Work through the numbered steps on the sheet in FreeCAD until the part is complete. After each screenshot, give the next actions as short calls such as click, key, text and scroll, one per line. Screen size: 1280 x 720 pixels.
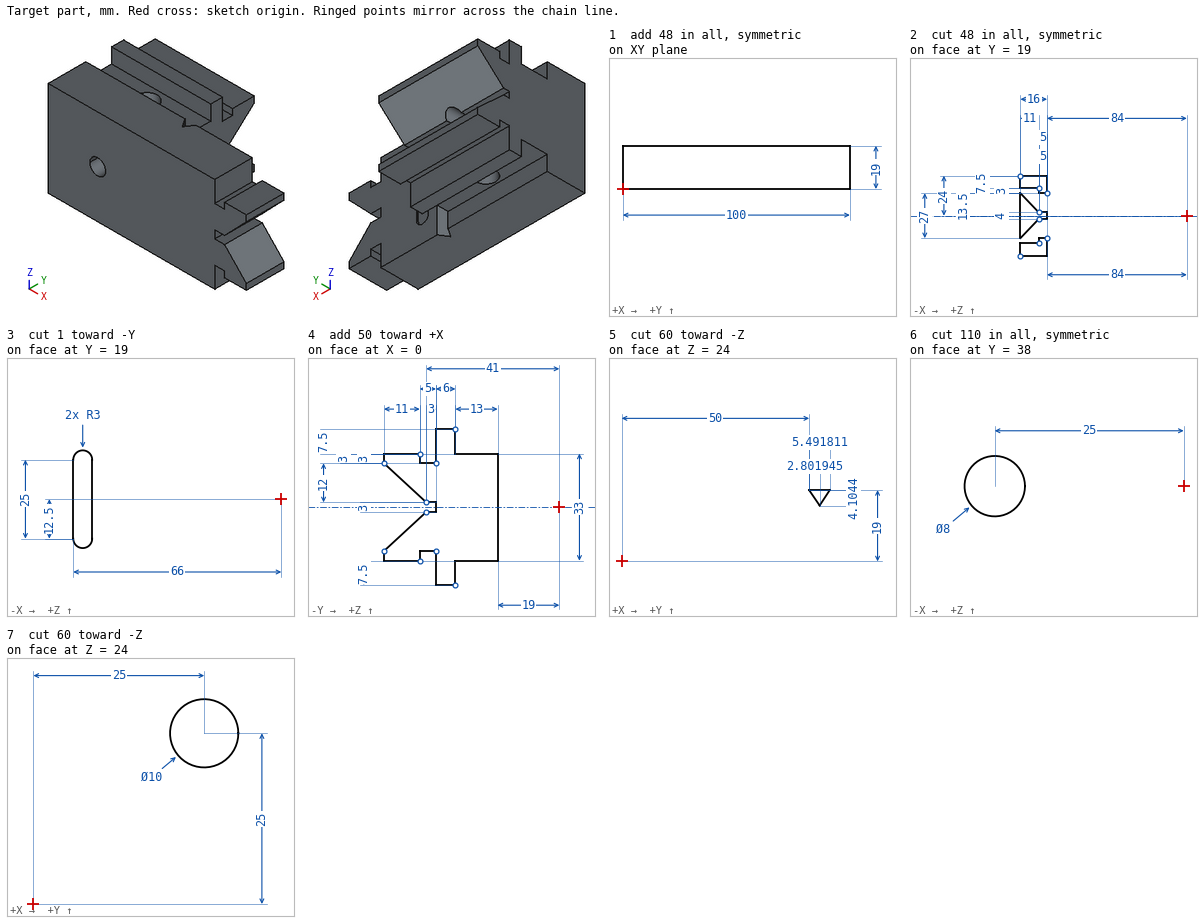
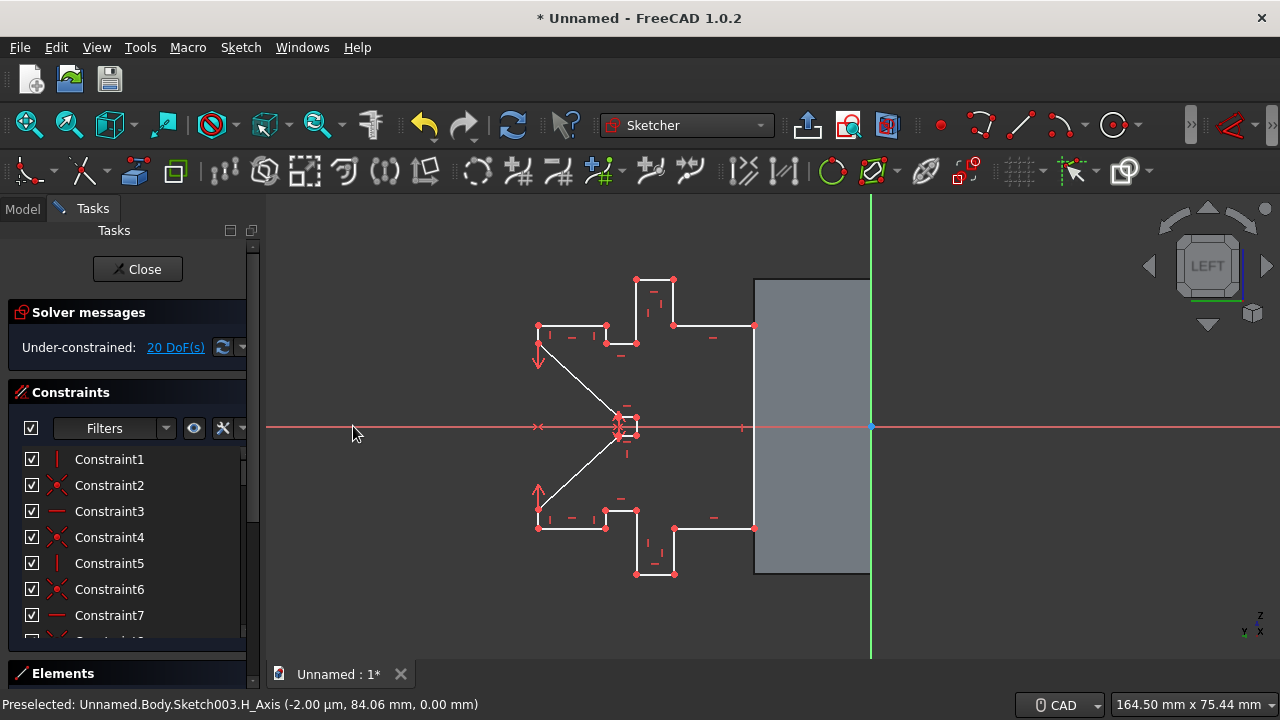
click(606, 326)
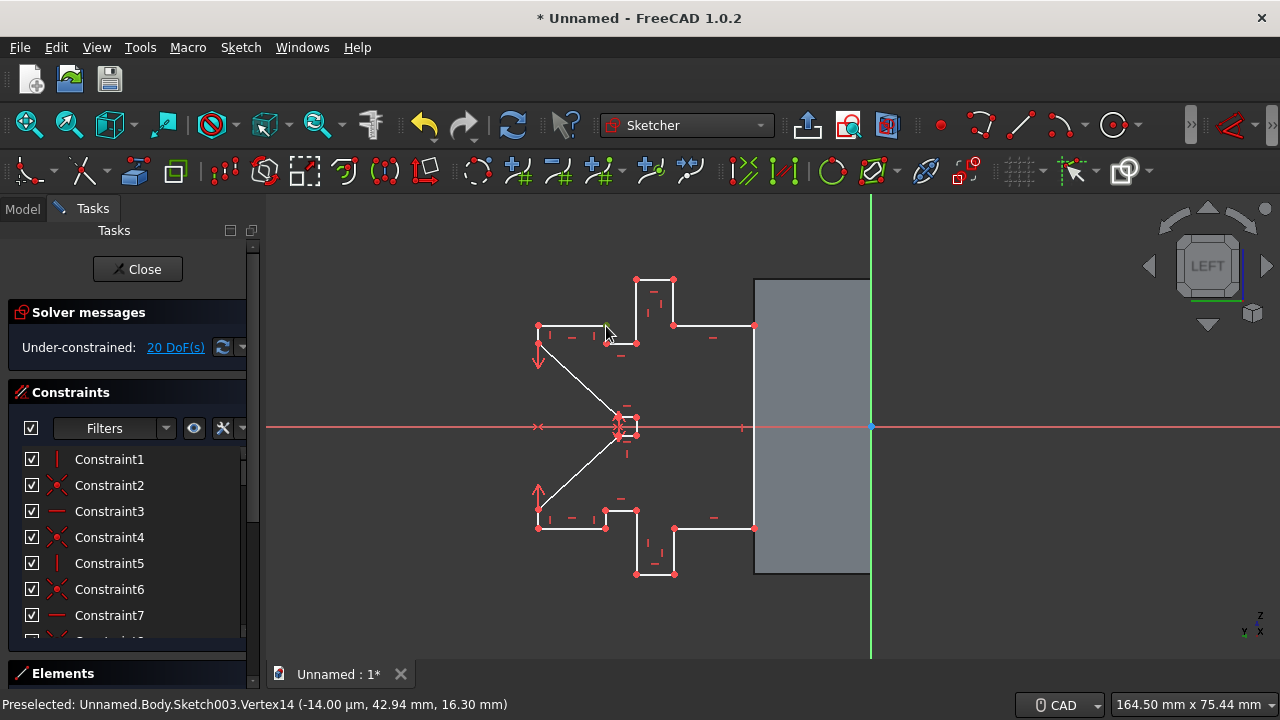
click(606, 529)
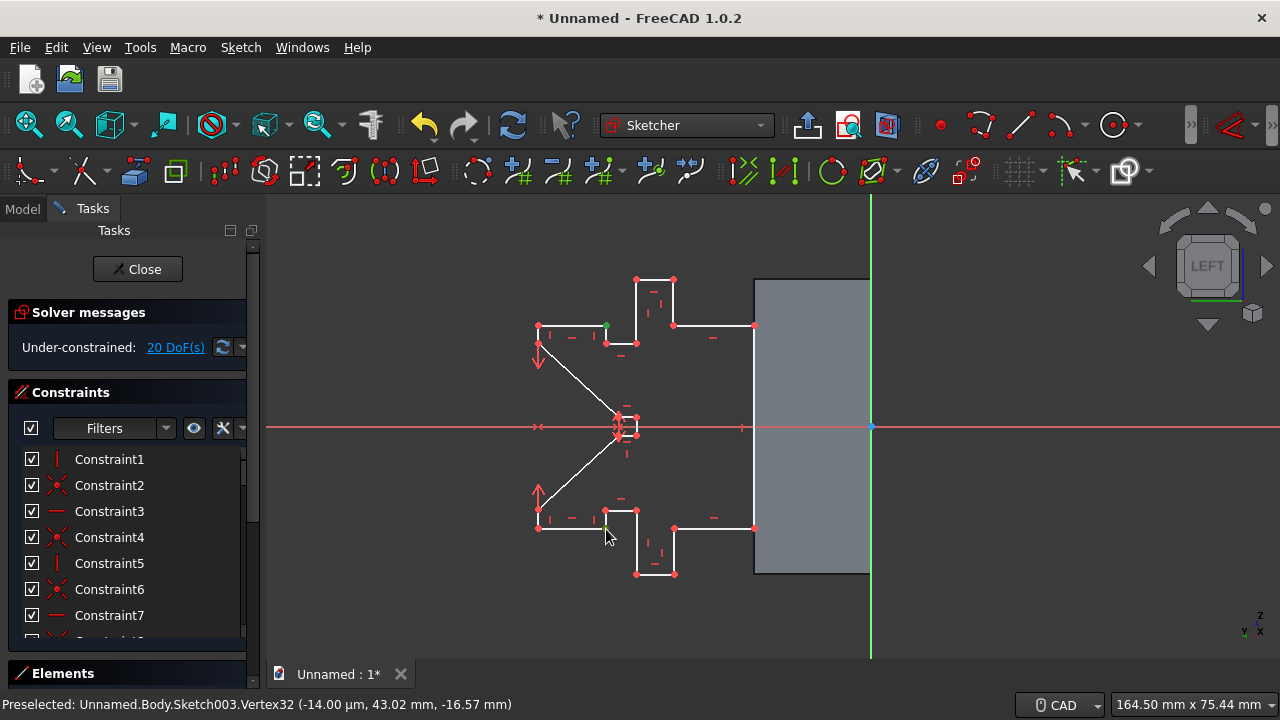
click(353, 426)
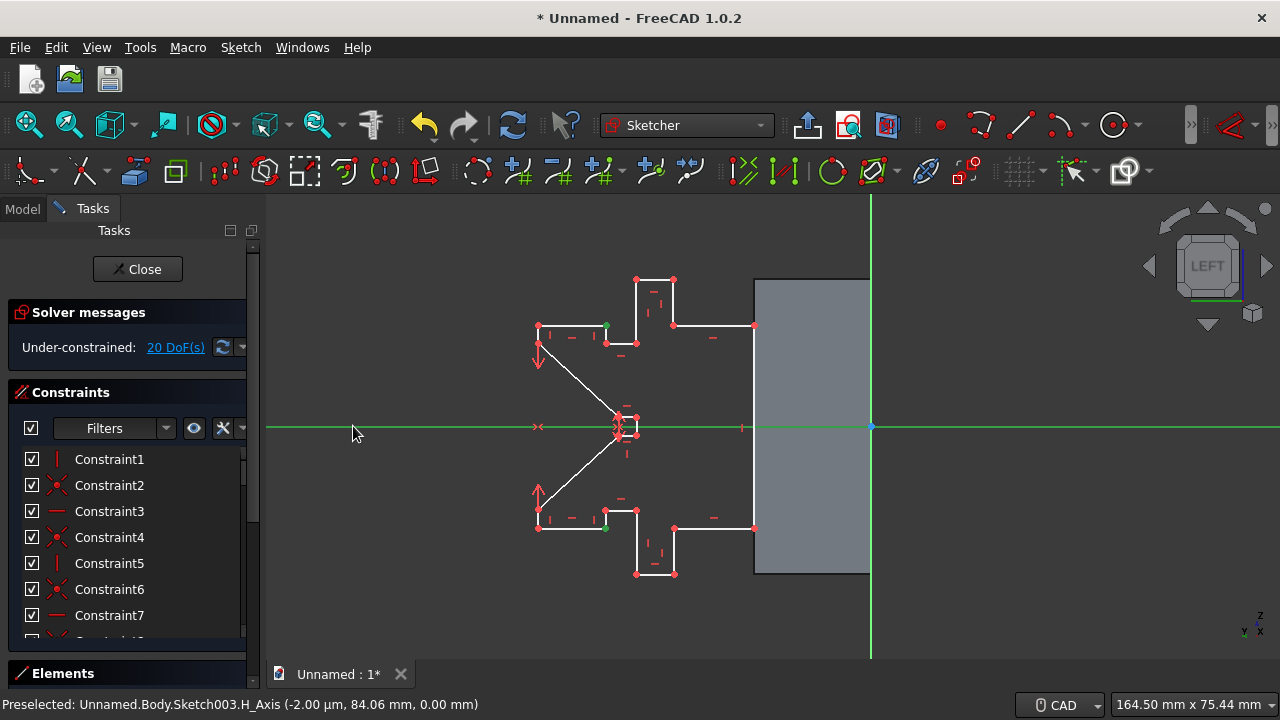
key(s)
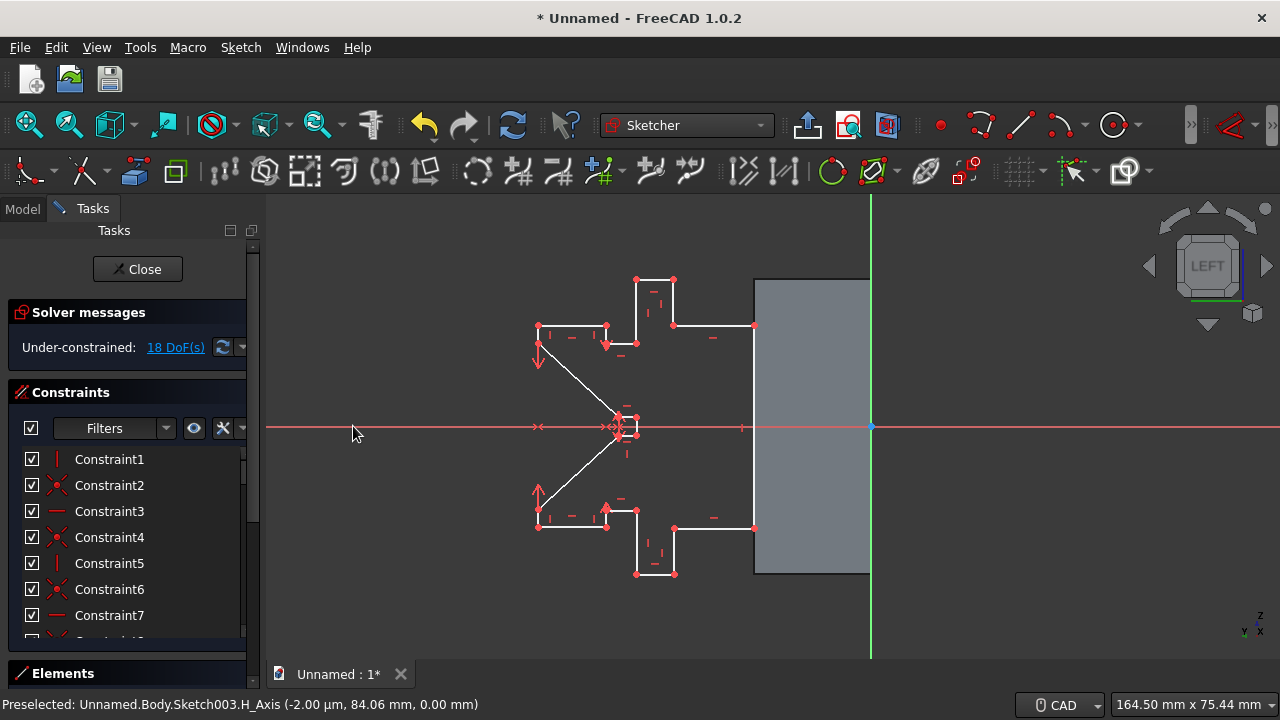
click(636, 344)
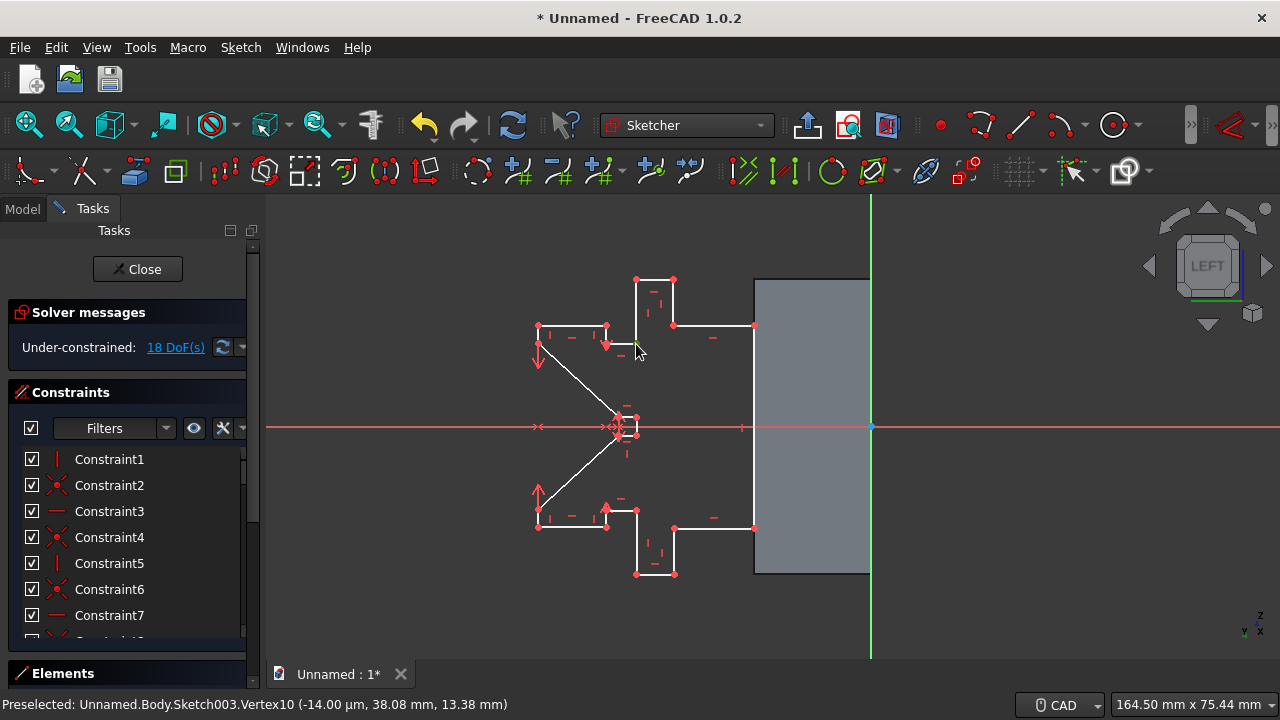
click(637, 511)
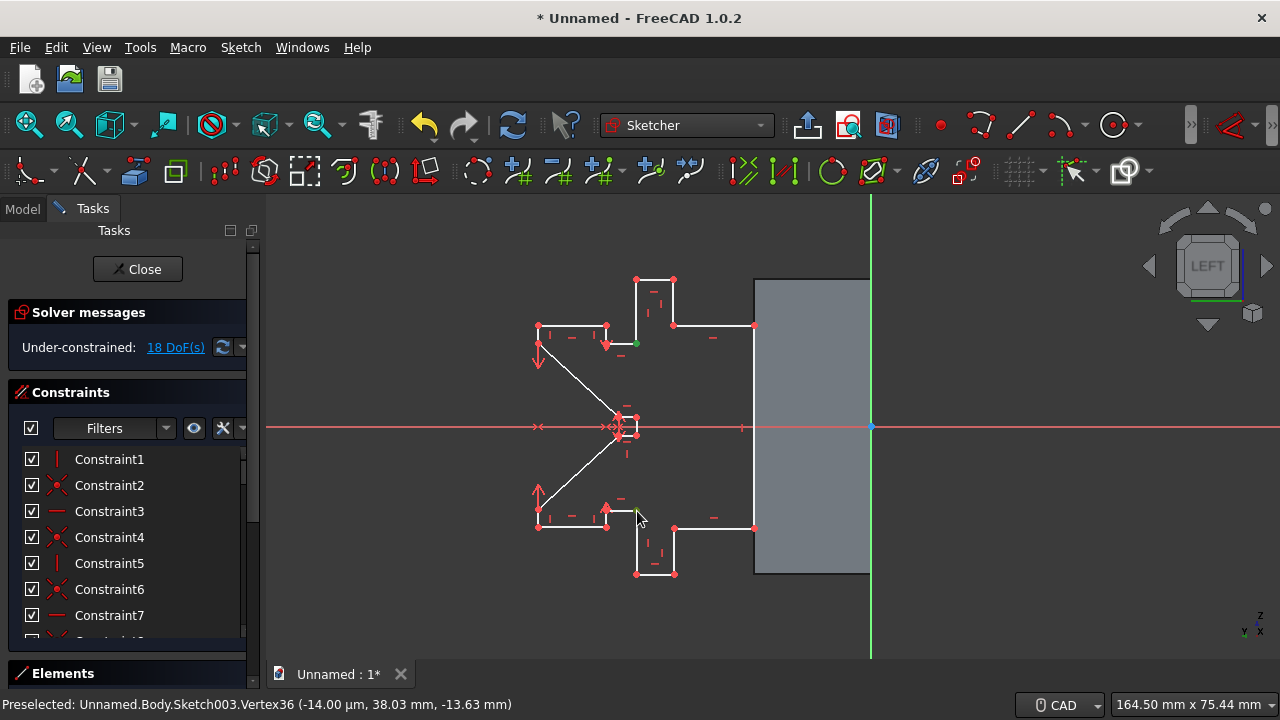
click(353, 426)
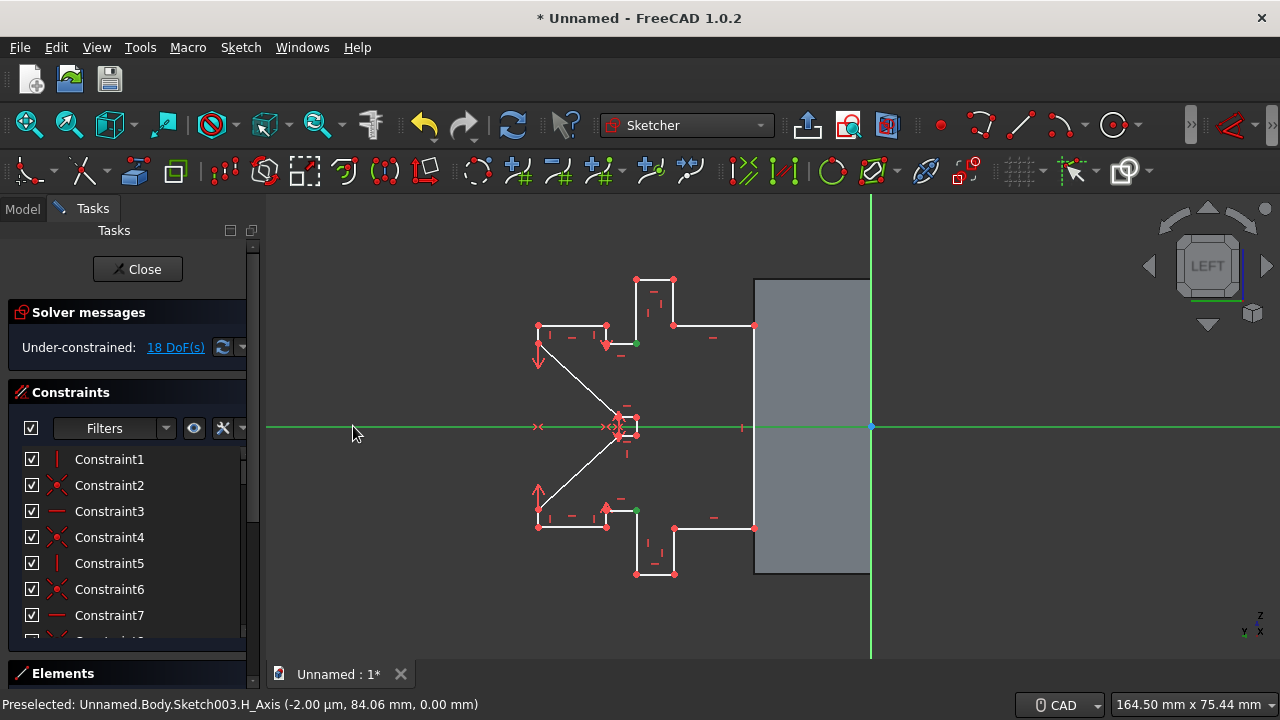
key(s)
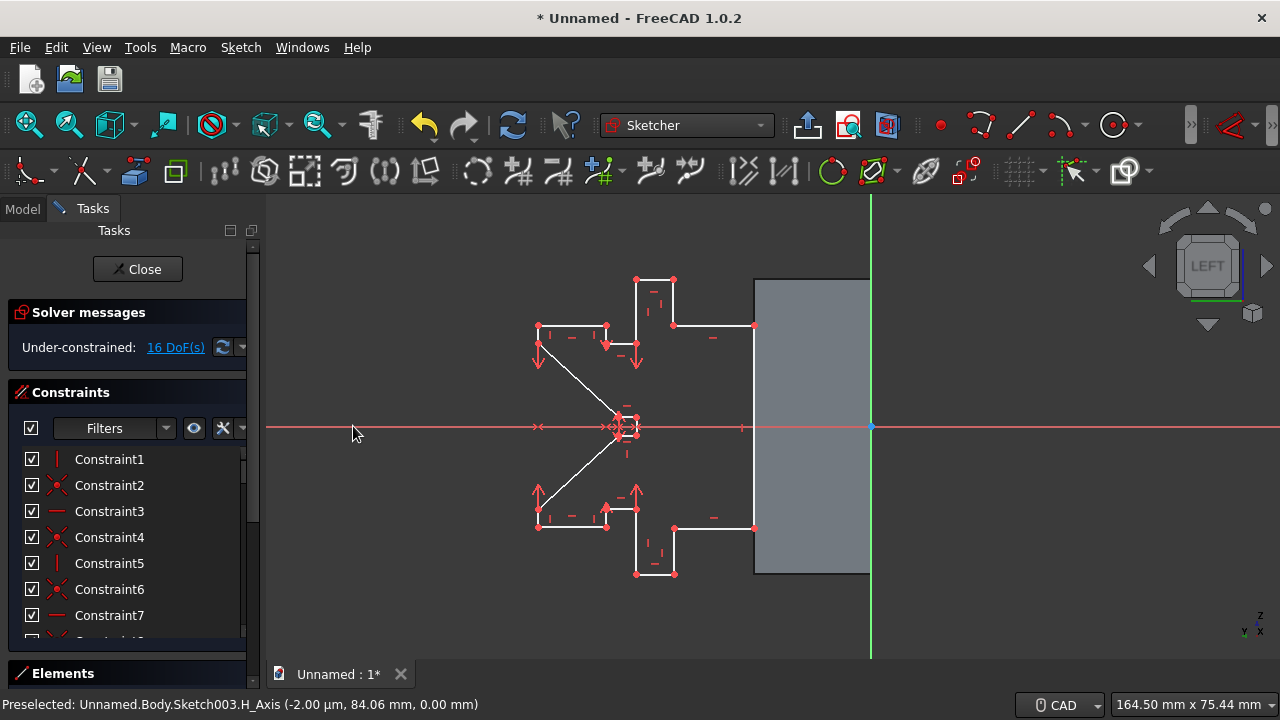
click(673, 280)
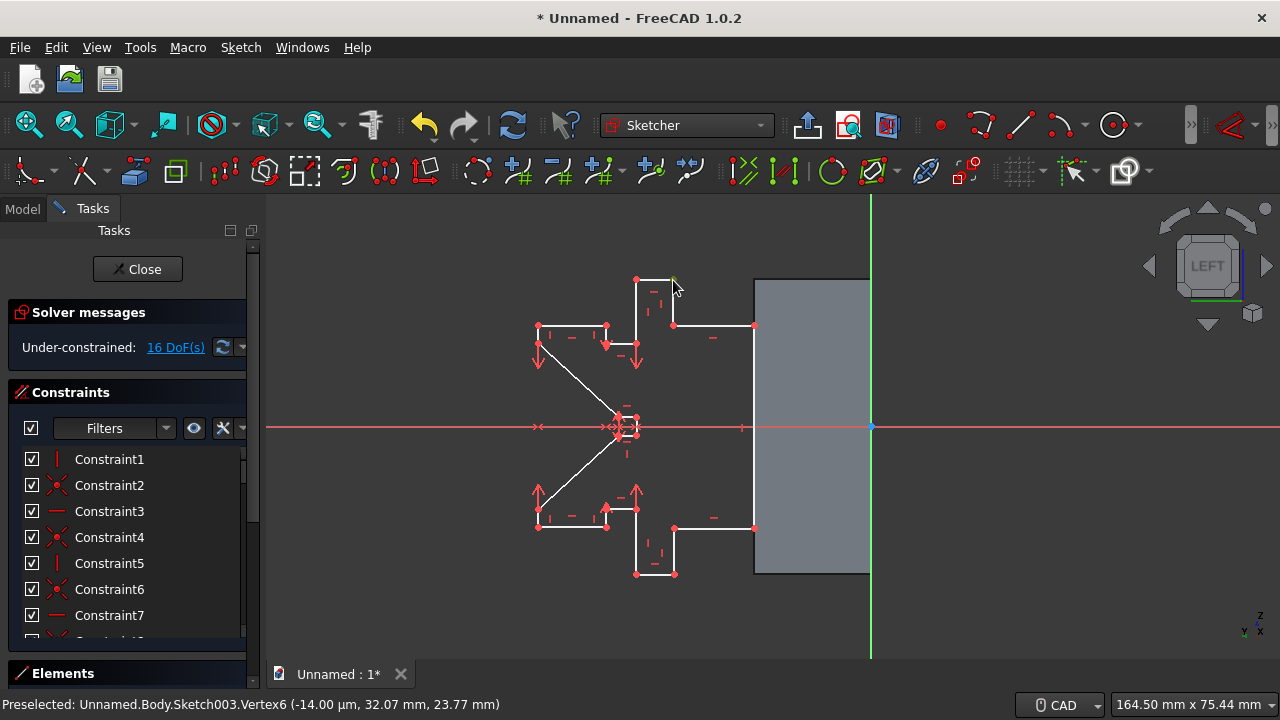
click(674, 575)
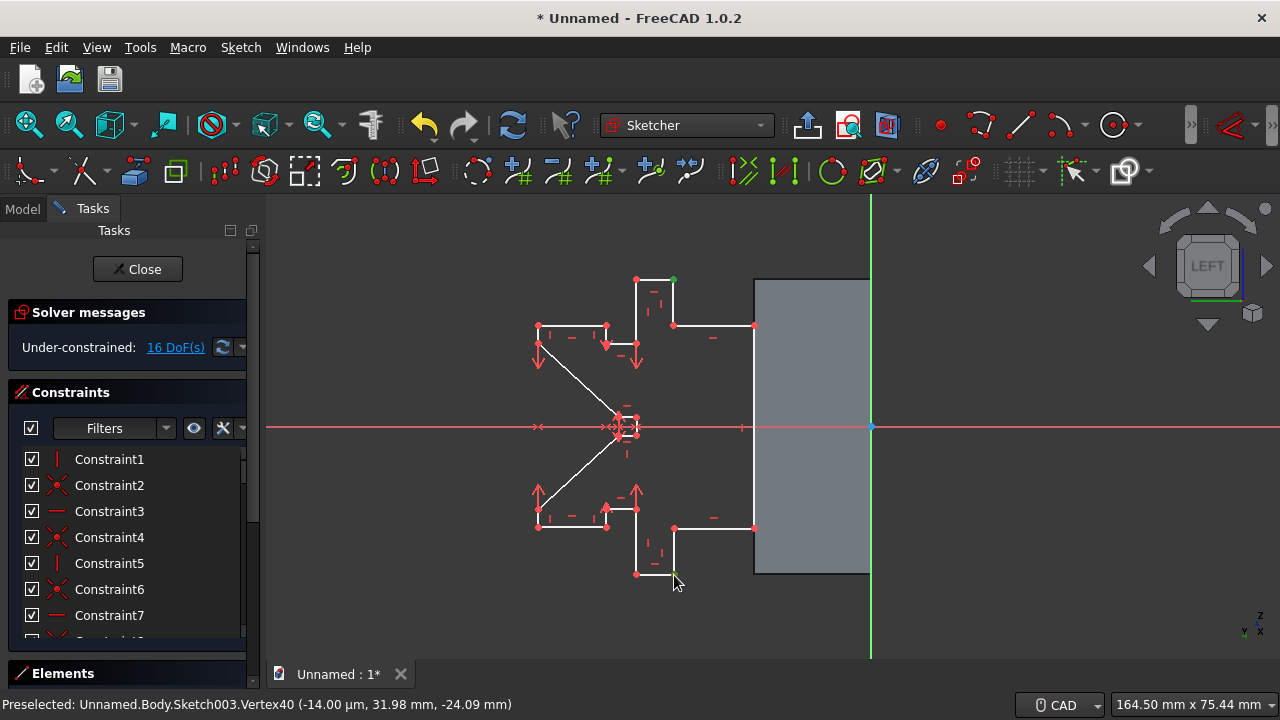
click(353, 426)